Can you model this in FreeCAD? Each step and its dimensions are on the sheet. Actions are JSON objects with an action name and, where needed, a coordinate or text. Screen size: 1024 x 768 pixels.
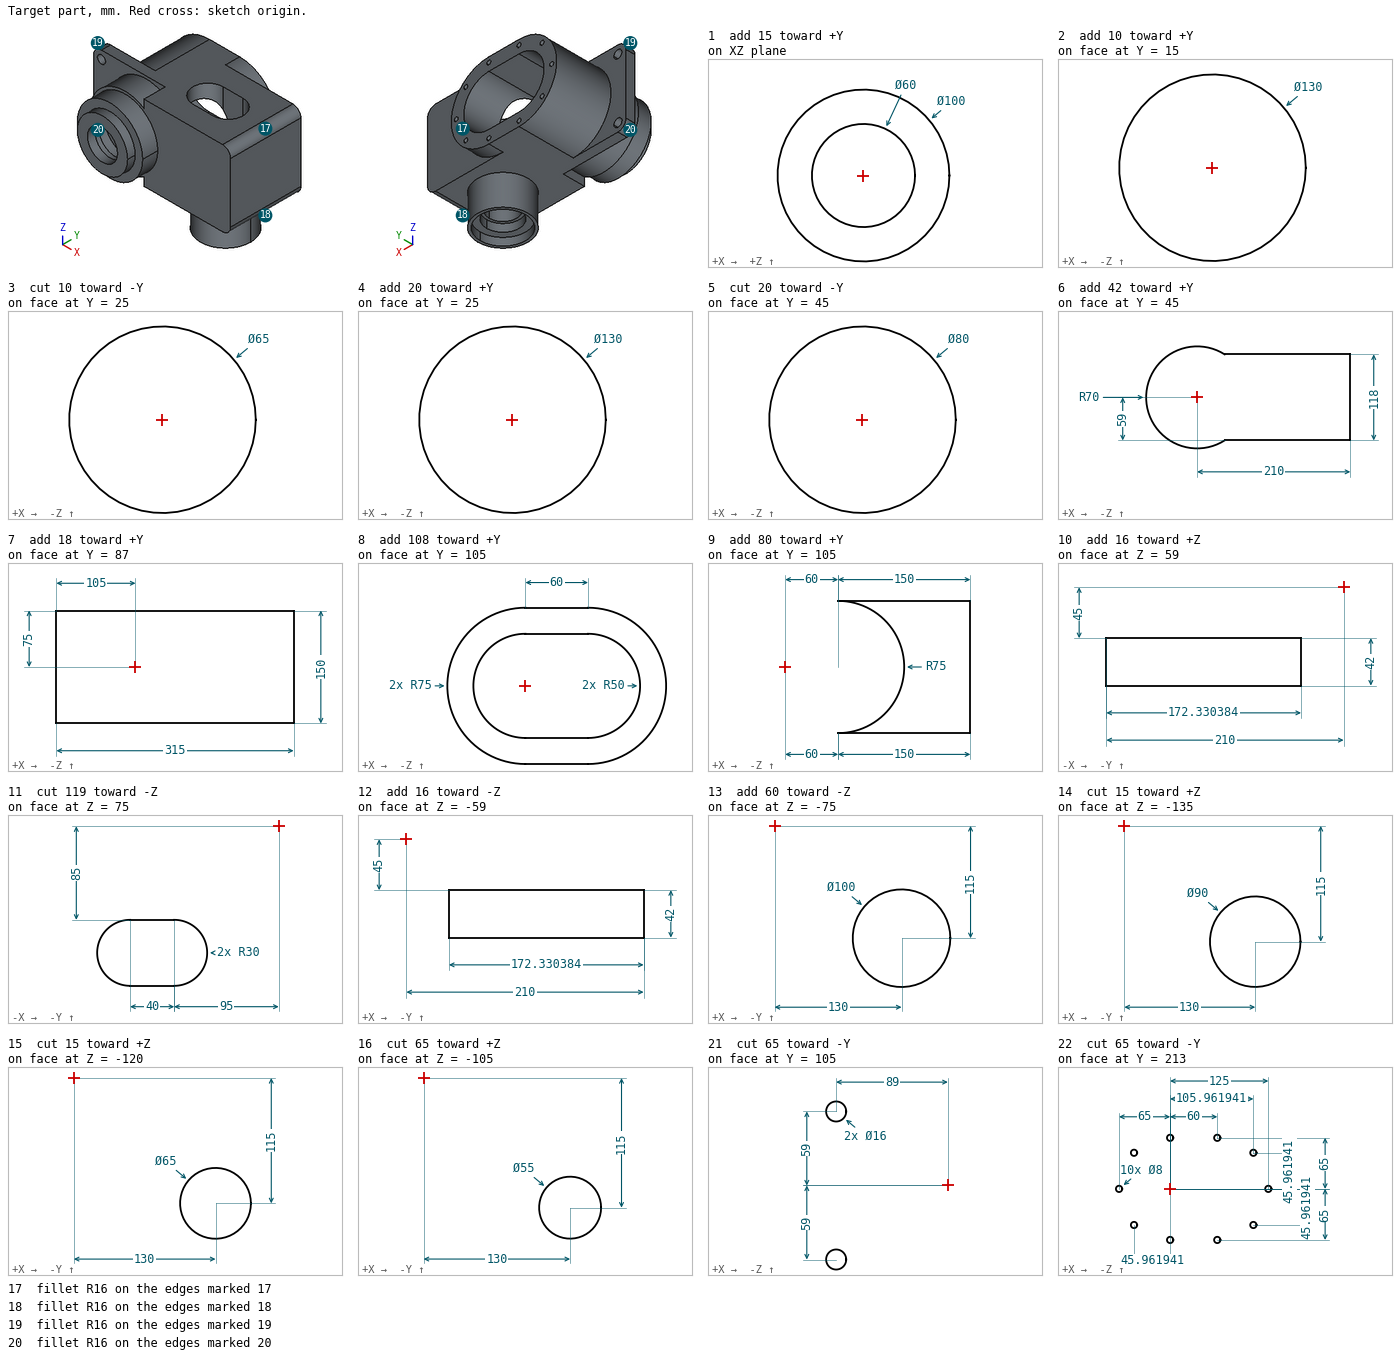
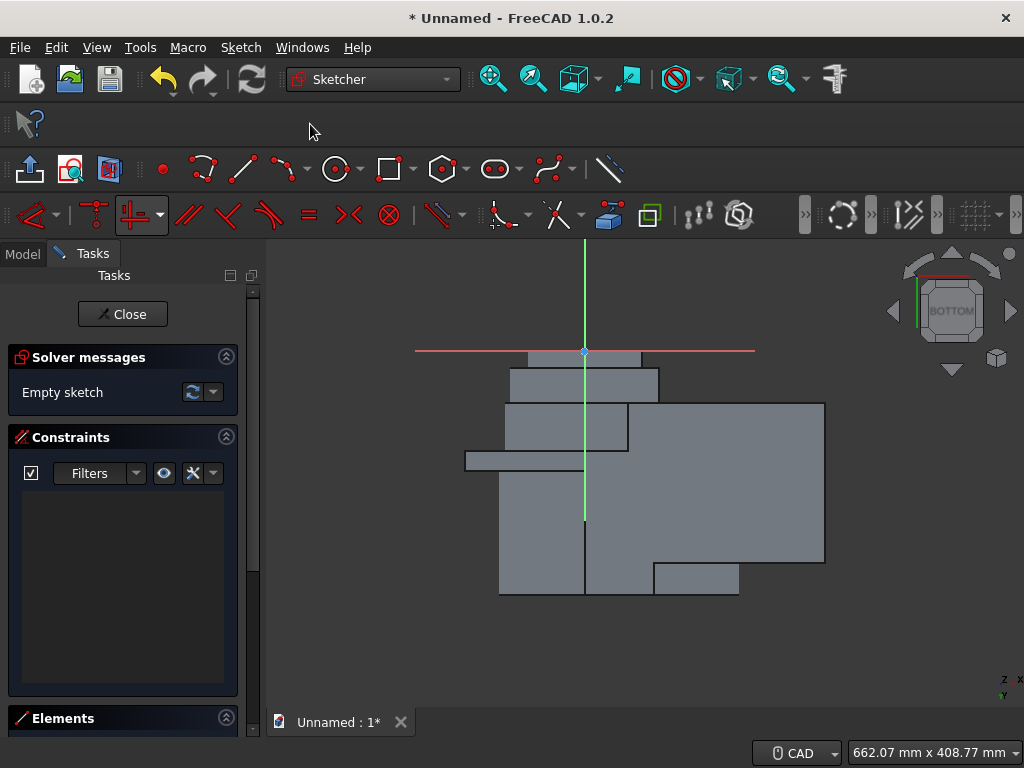
{"action": "scroll", "coordinate": [859, 390], "scroll_direction": "up", "scroll_amount": 2}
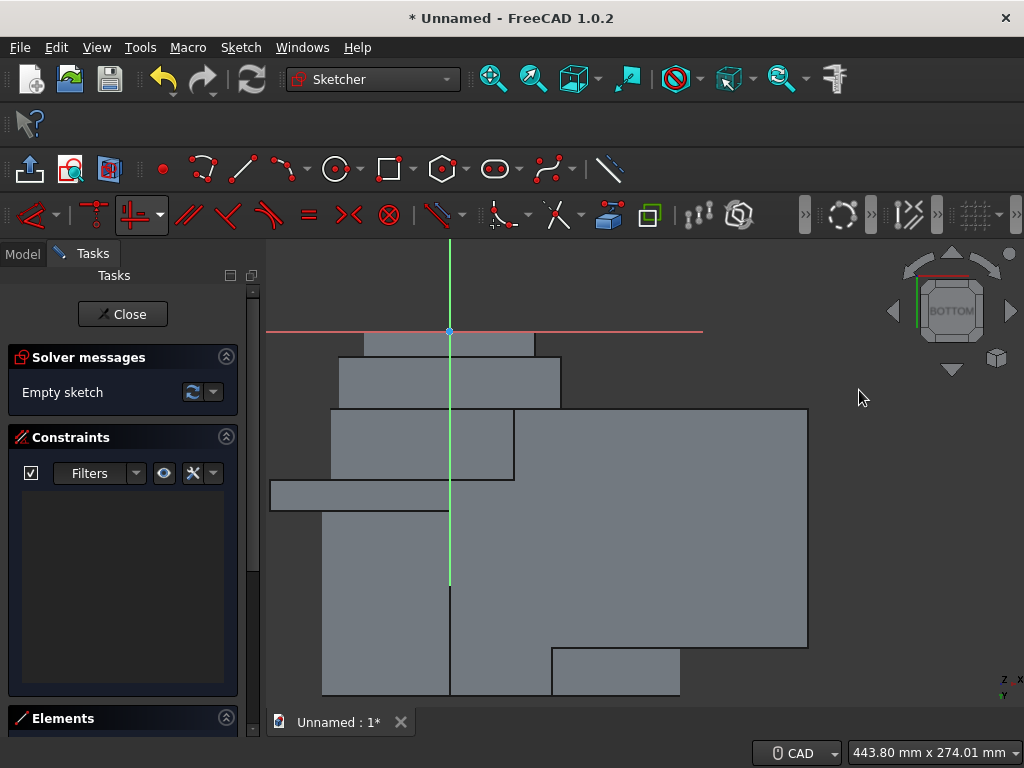
{"action": "left_click", "coordinate": [336, 170]}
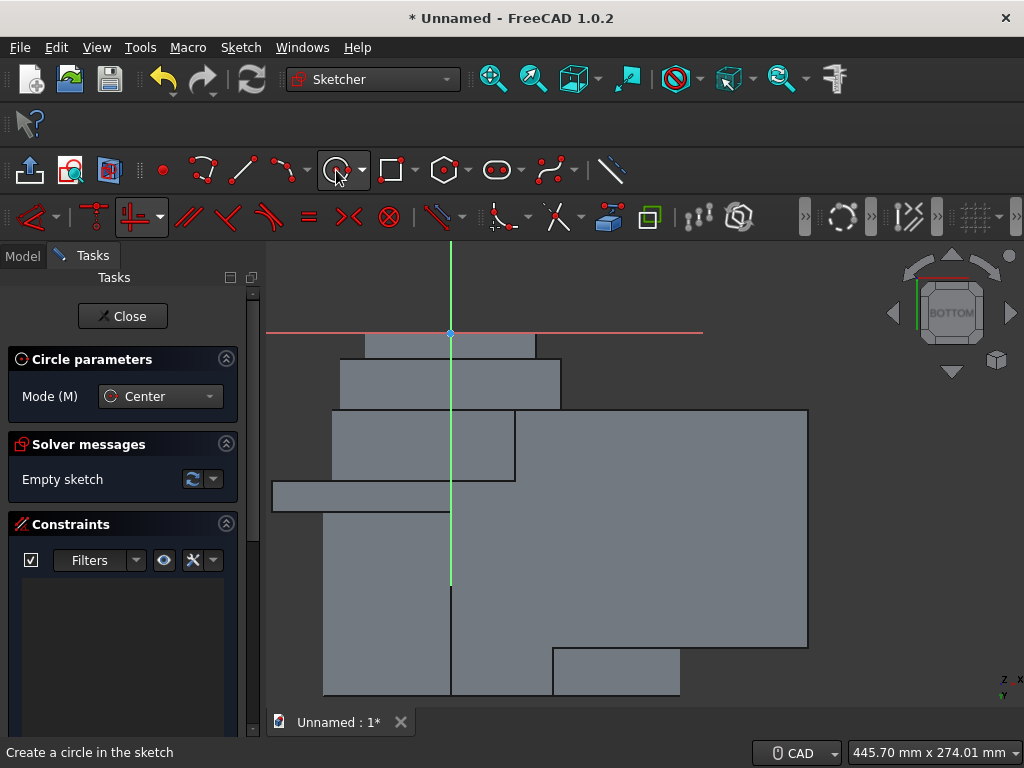
{"action": "left_click", "coordinate": [672, 529]}
{"action": "mouse_move", "coordinate": [732, 469]}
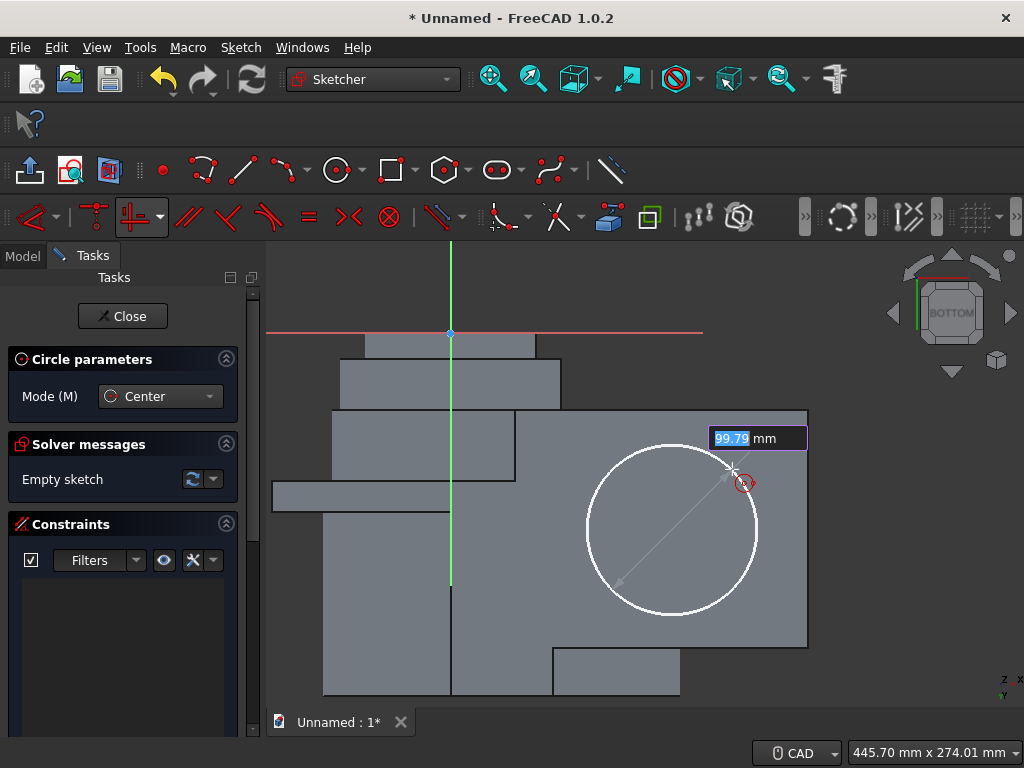
{"action": "type", "text": "100"}
{"action": "key", "text": "Return"}
{"action": "key", "text": "Escape"}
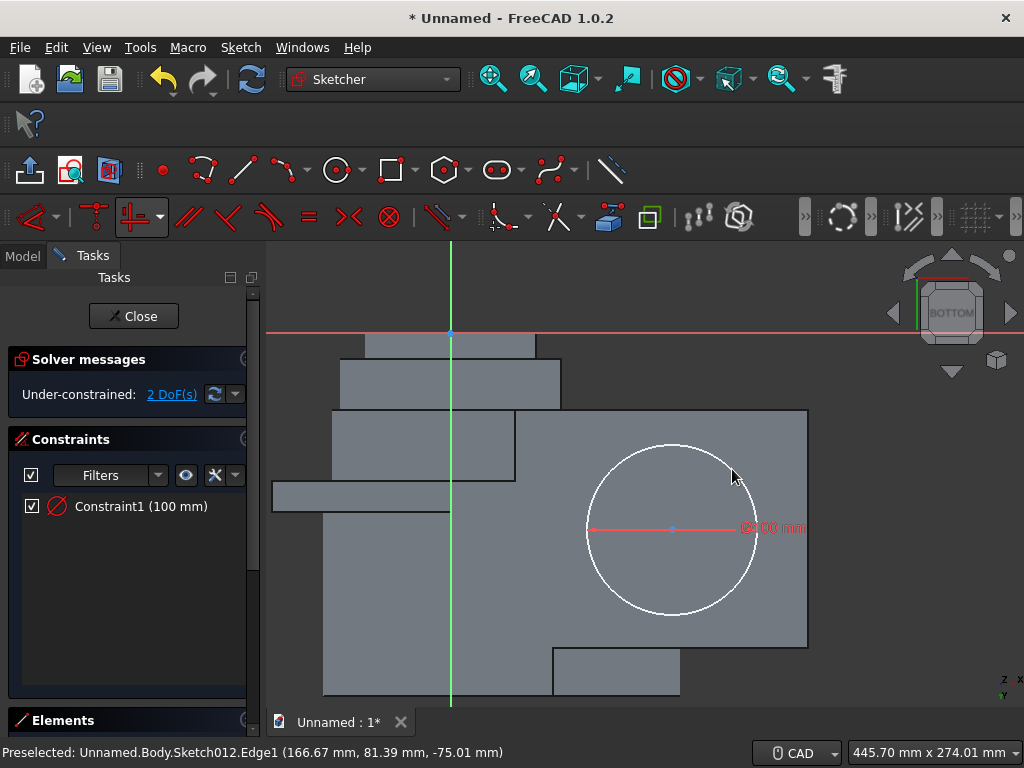
{"action": "left_click", "coordinate": [32, 218]}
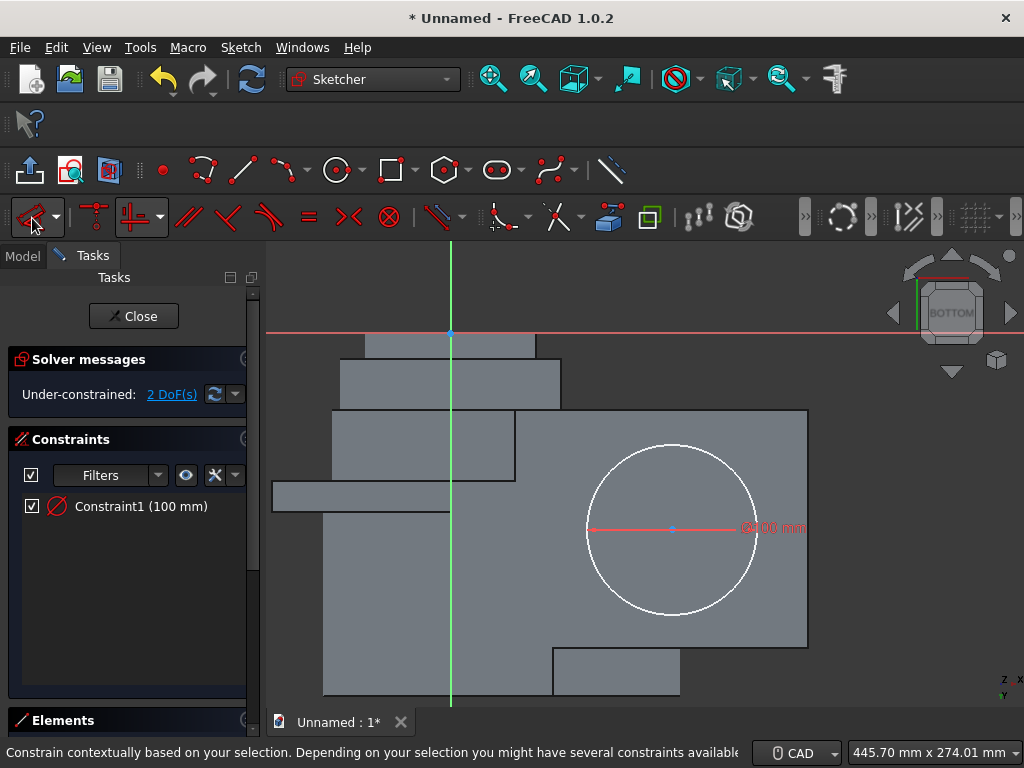
{"action": "left_click", "coordinate": [672, 530]}
{"action": "left_click", "coordinate": [561, 299]}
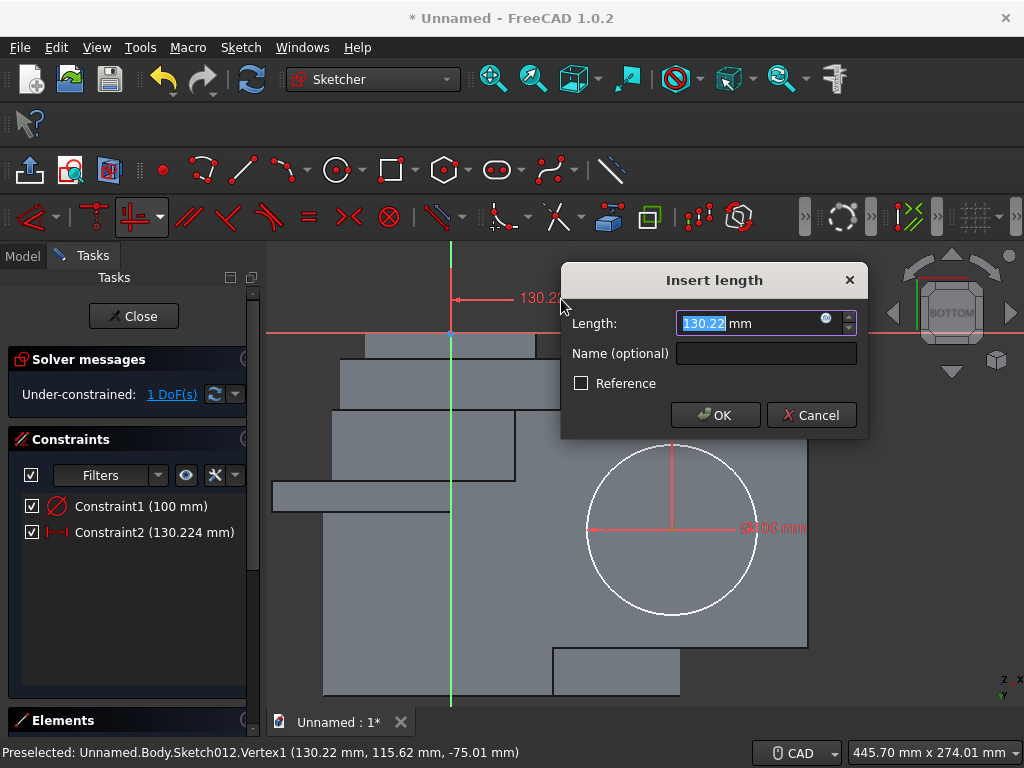
{"action": "type", "text": "130"}
{"action": "key", "text": "Return"}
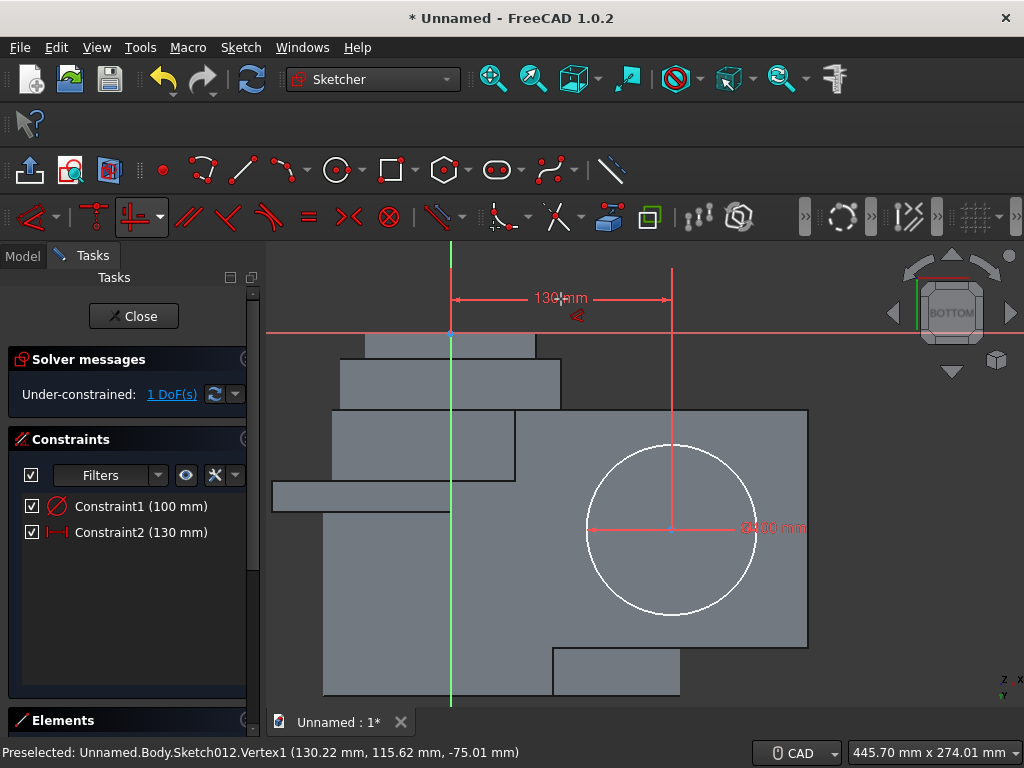
{"action": "left_click", "coordinate": [672, 530]}
{"action": "left_click", "coordinate": [417, 432]}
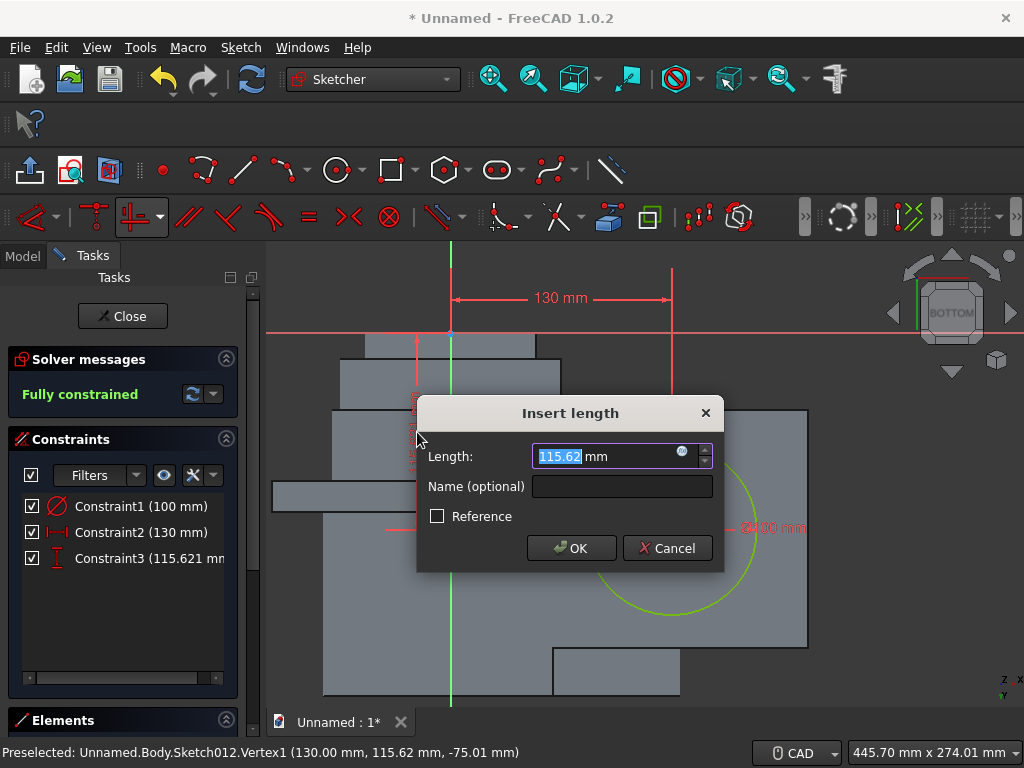
{"action": "type", "text": "115"}
{"action": "key", "text": "Return"}
{"action": "key", "text": "Escape"}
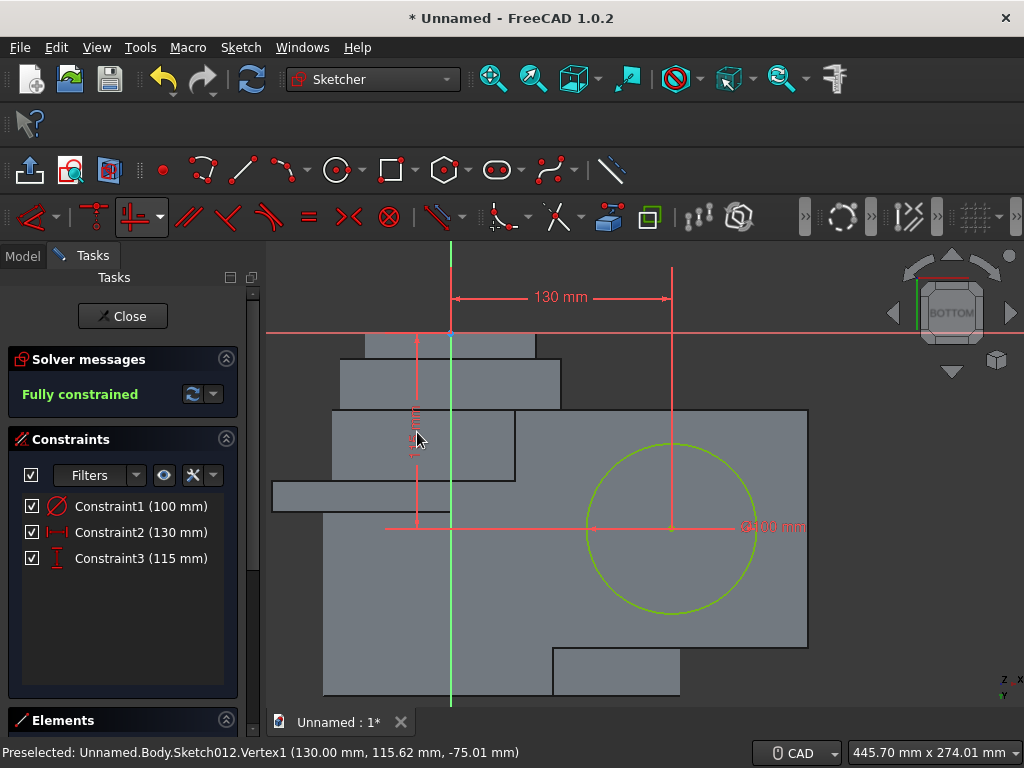
{"action": "left_click", "coordinate": [123, 316]}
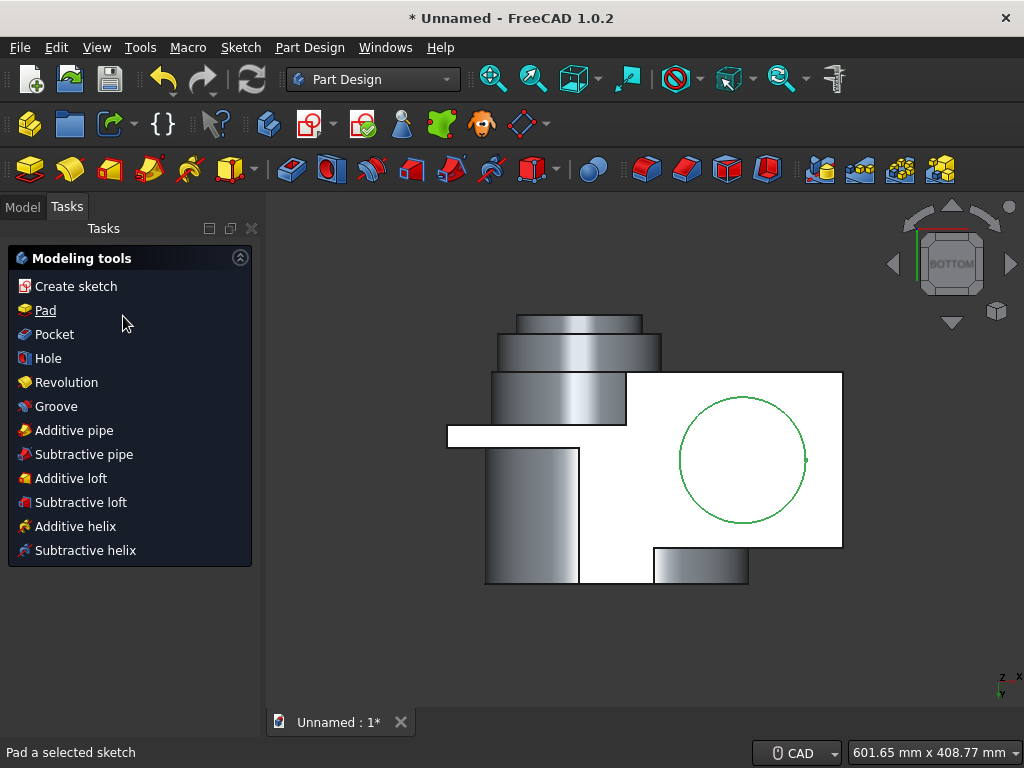
{"action": "left_click", "coordinate": [30, 170]}